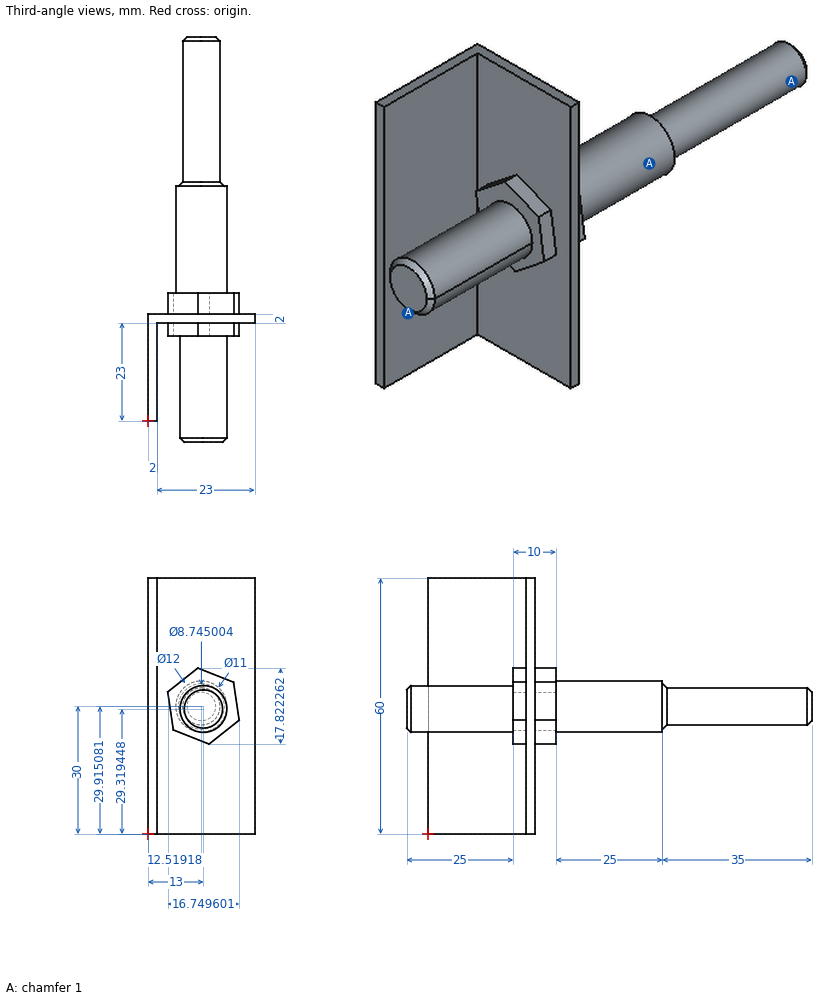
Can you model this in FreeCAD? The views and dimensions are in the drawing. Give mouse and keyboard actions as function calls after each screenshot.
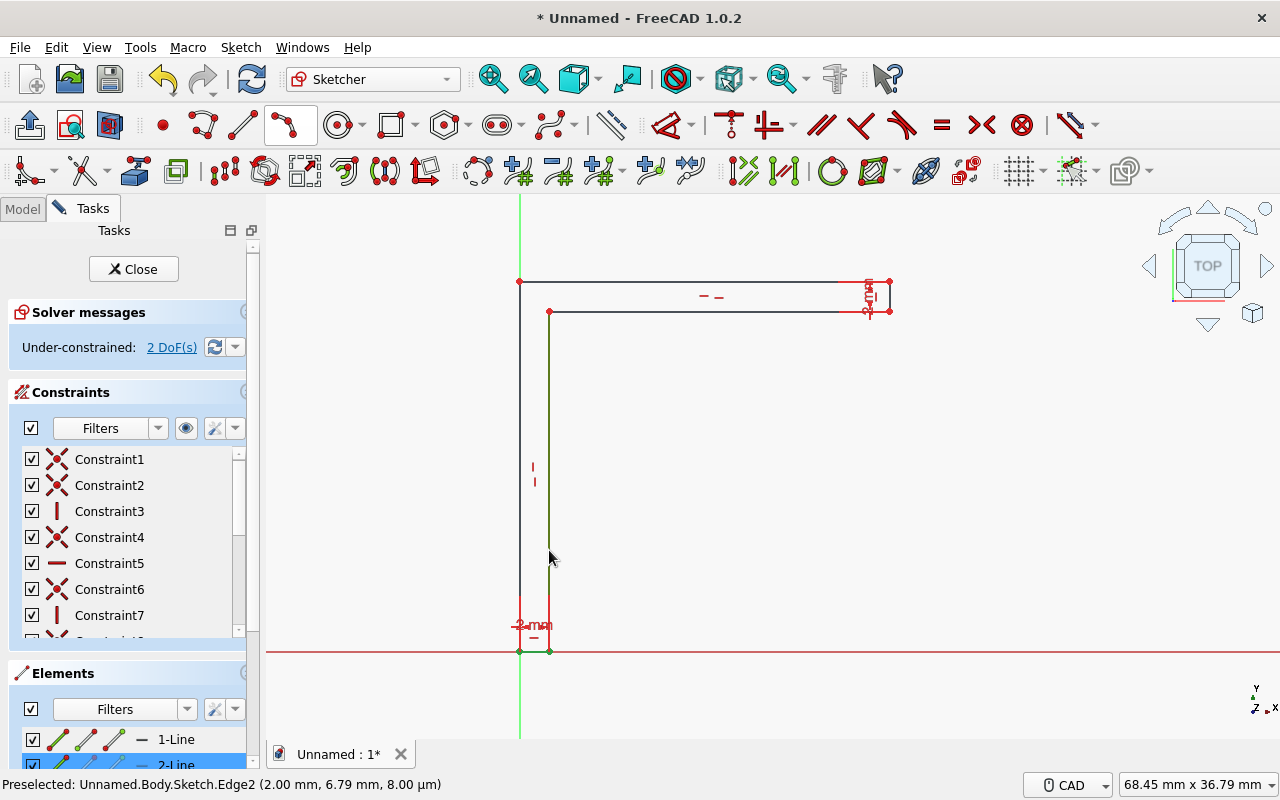
key(i)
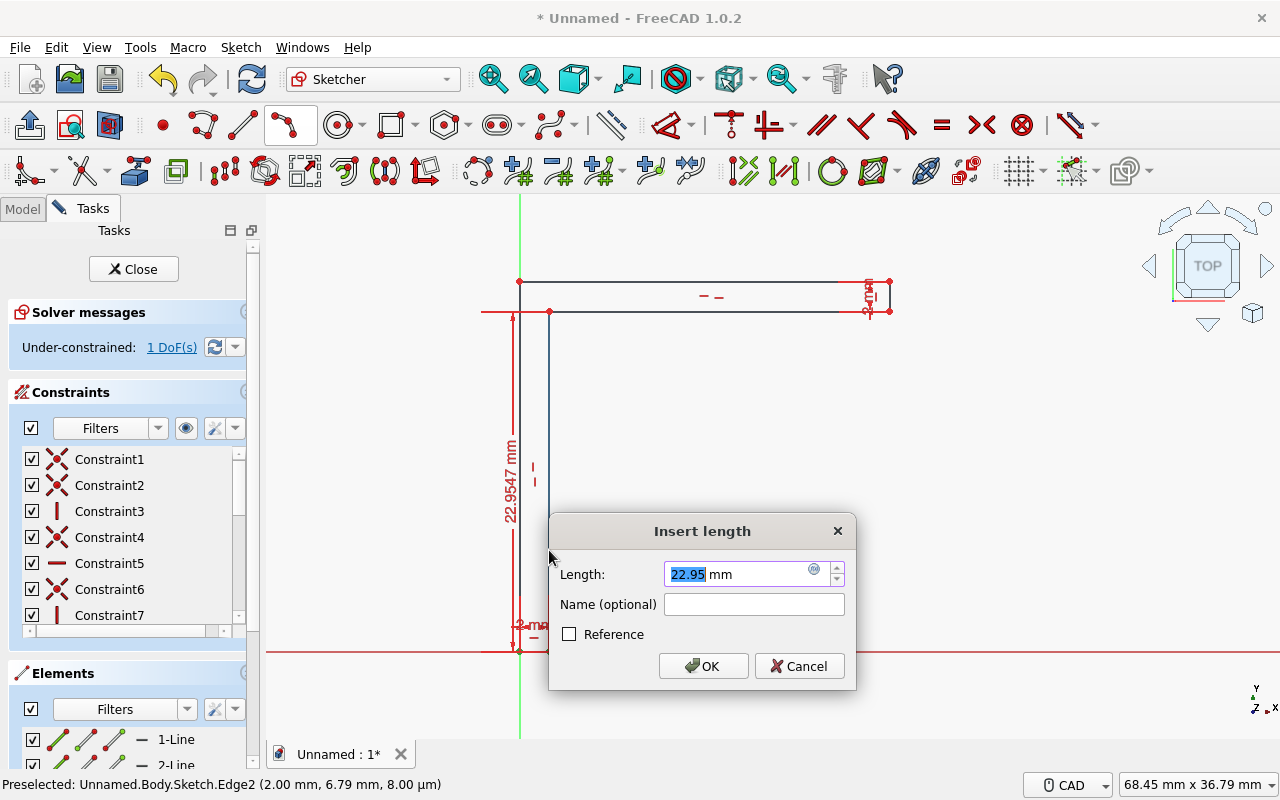
text(23)
key(Return)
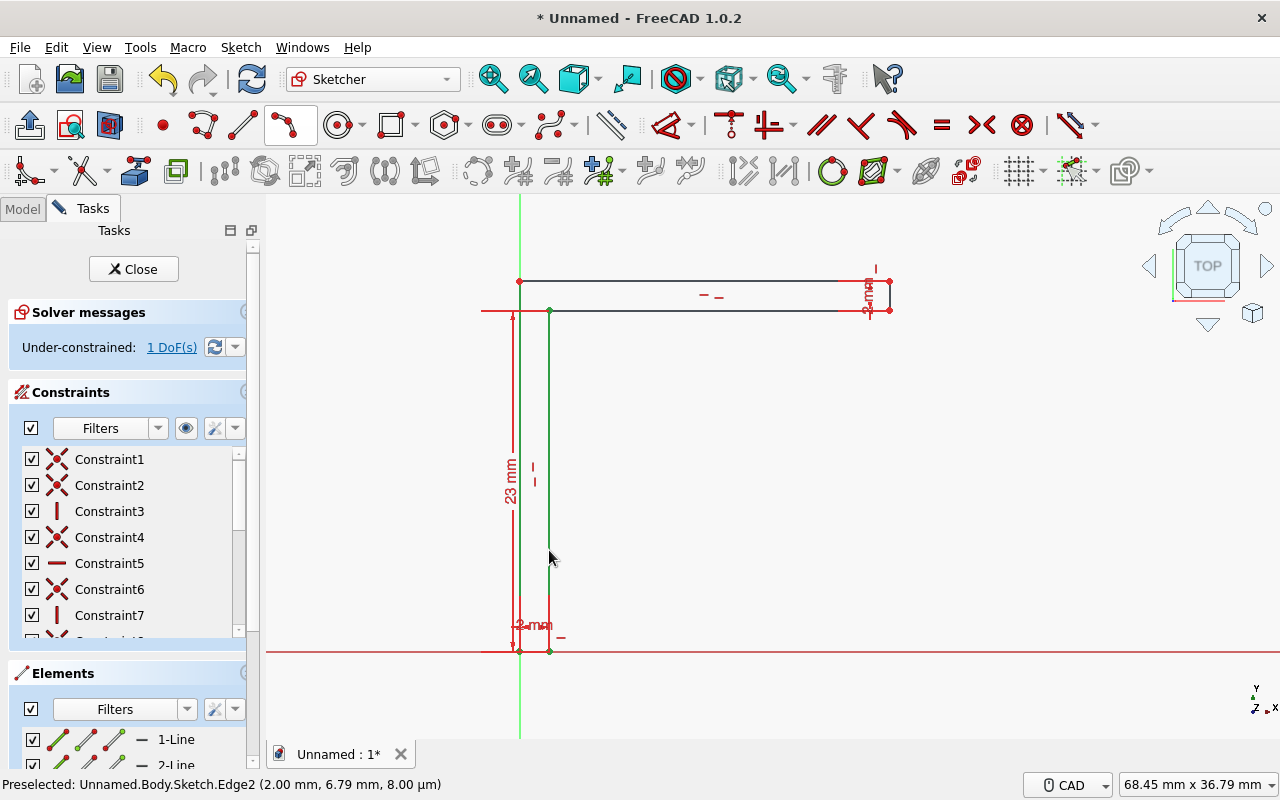
click(651, 311)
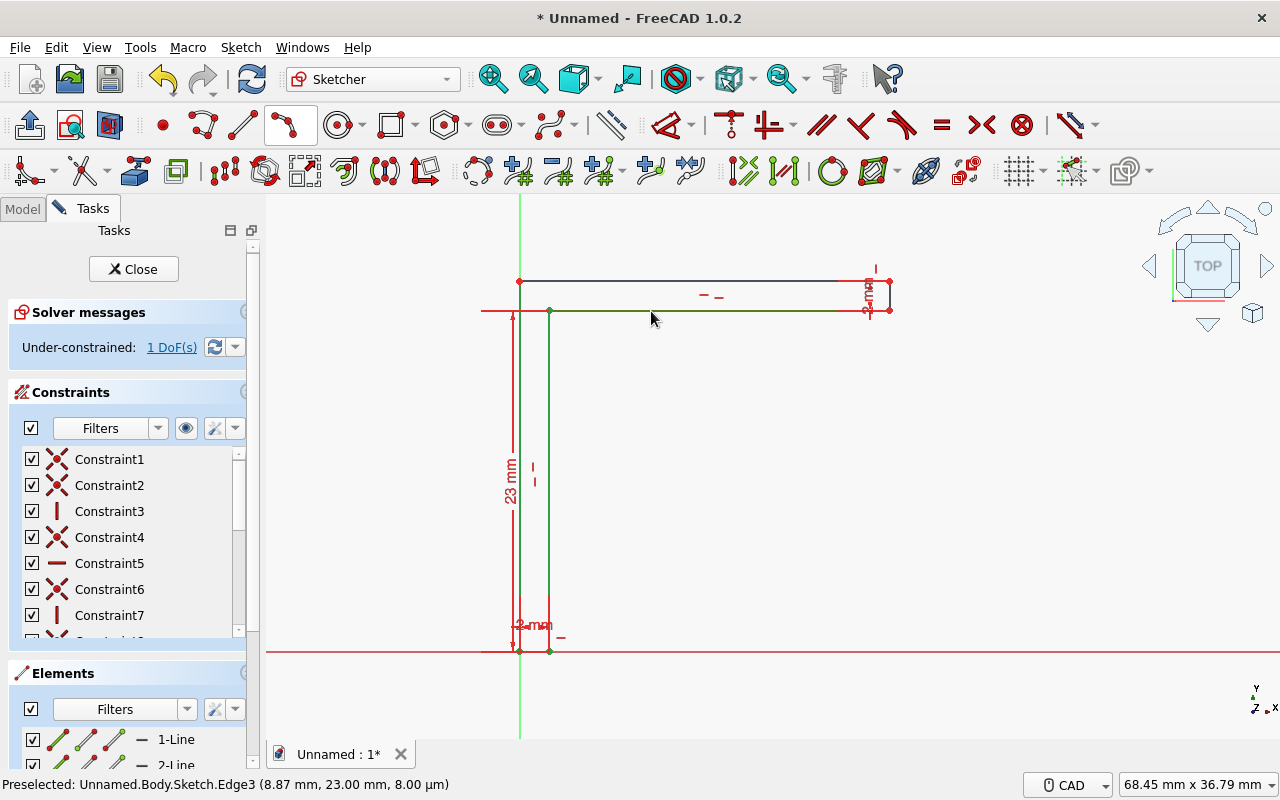
click(694, 126)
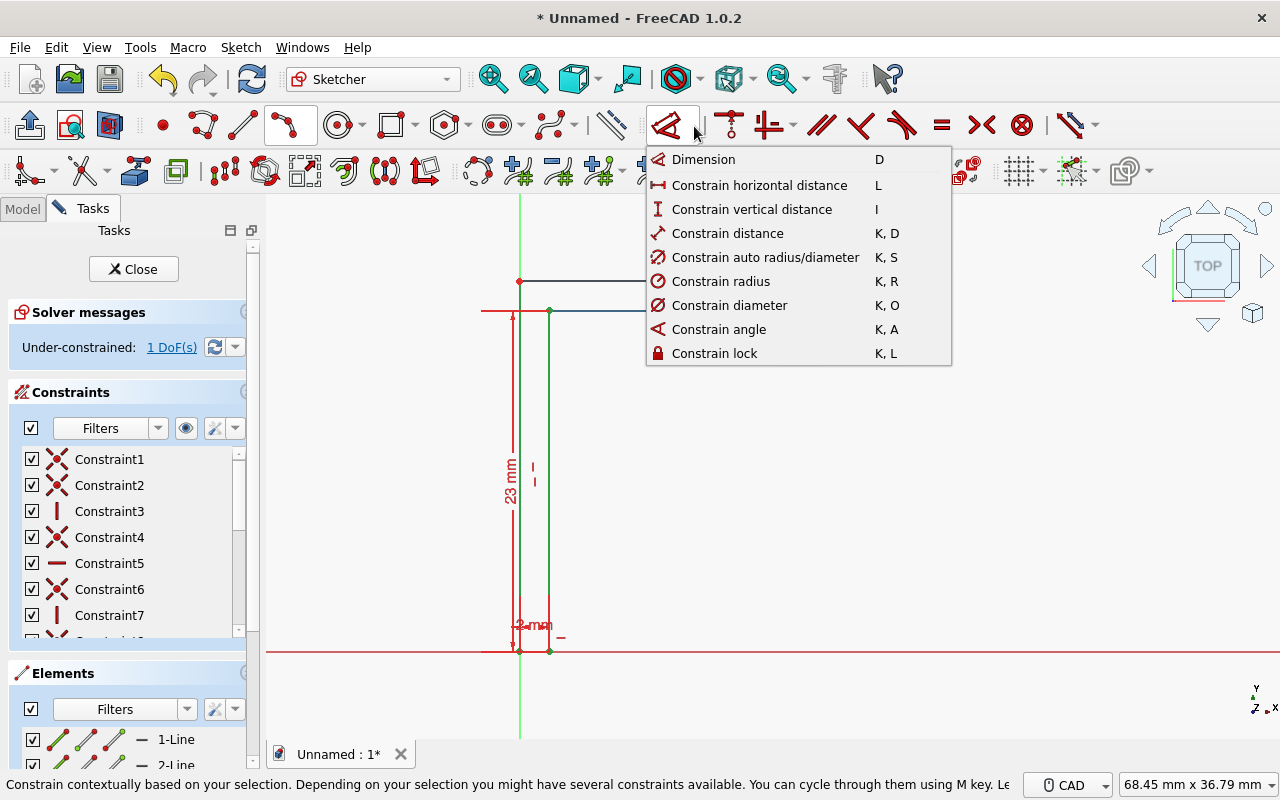
click(799, 185)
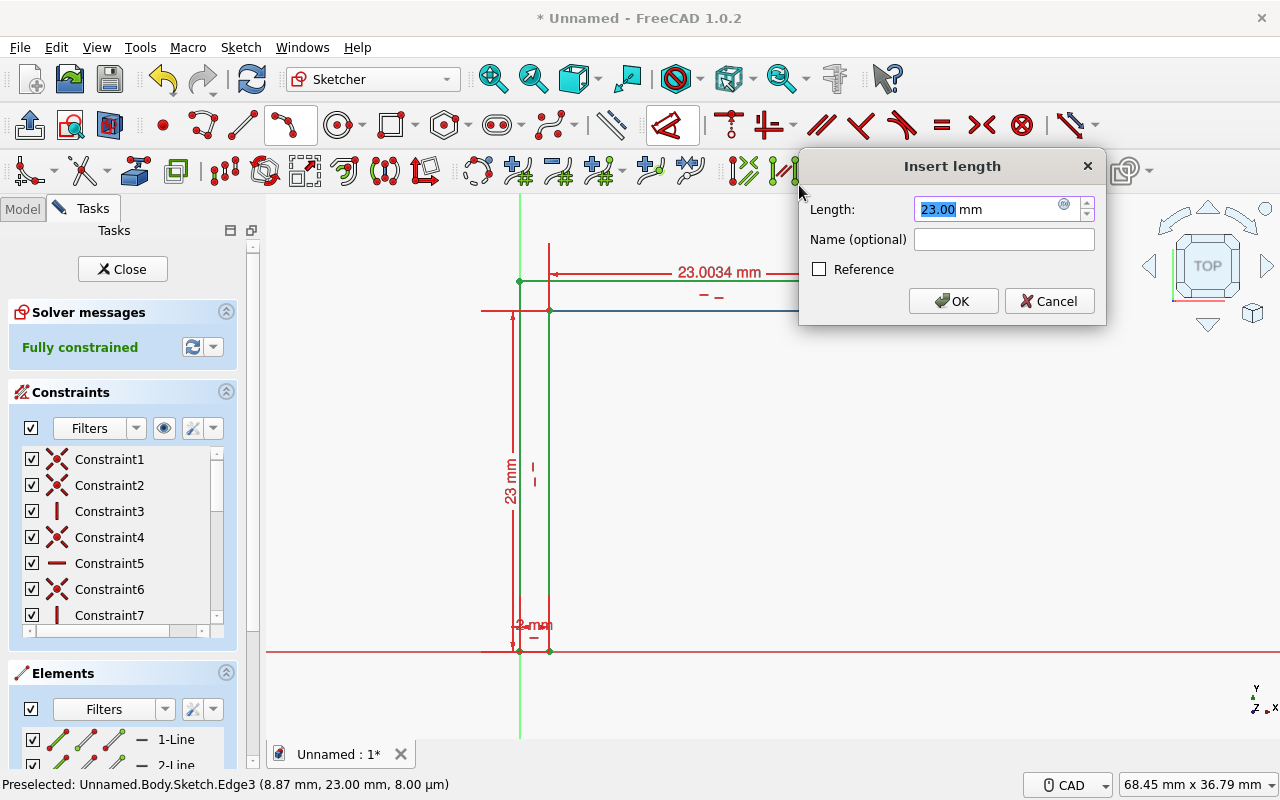
text(23)
key(Return)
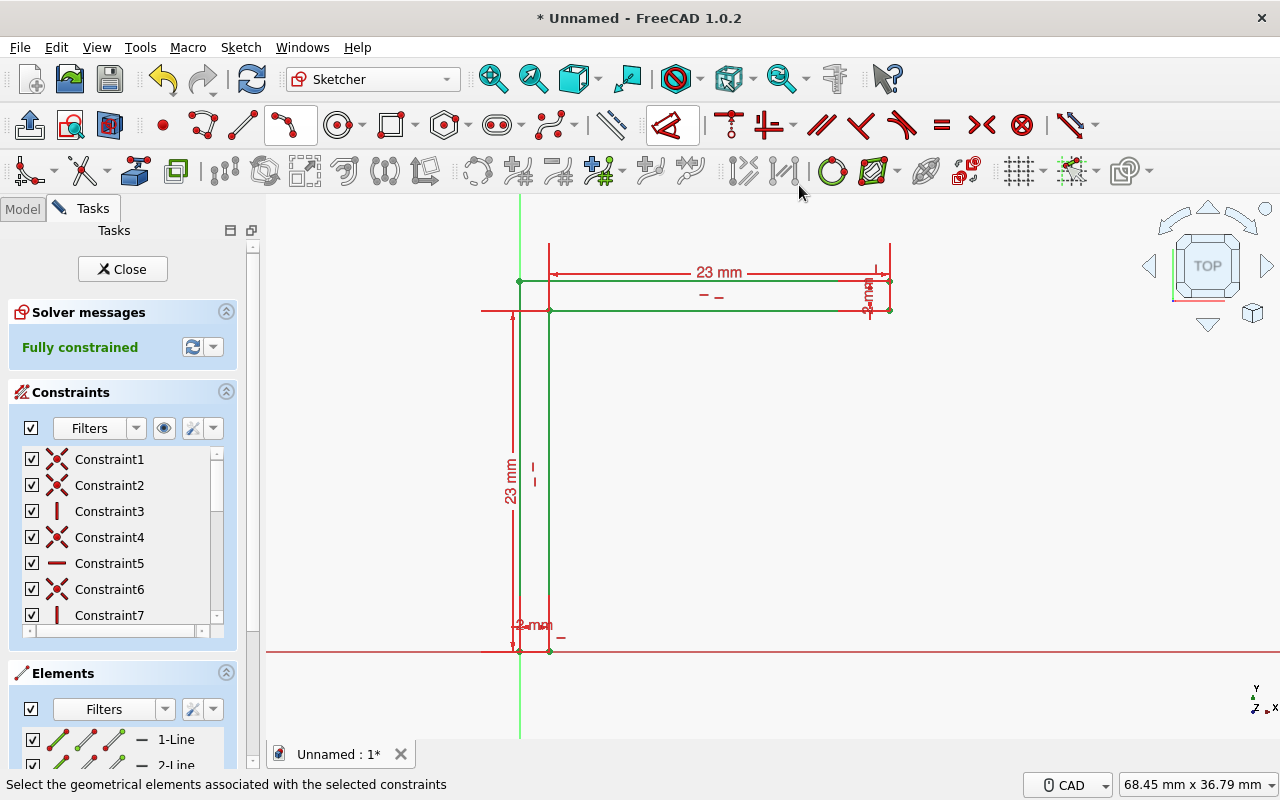
click(123, 269)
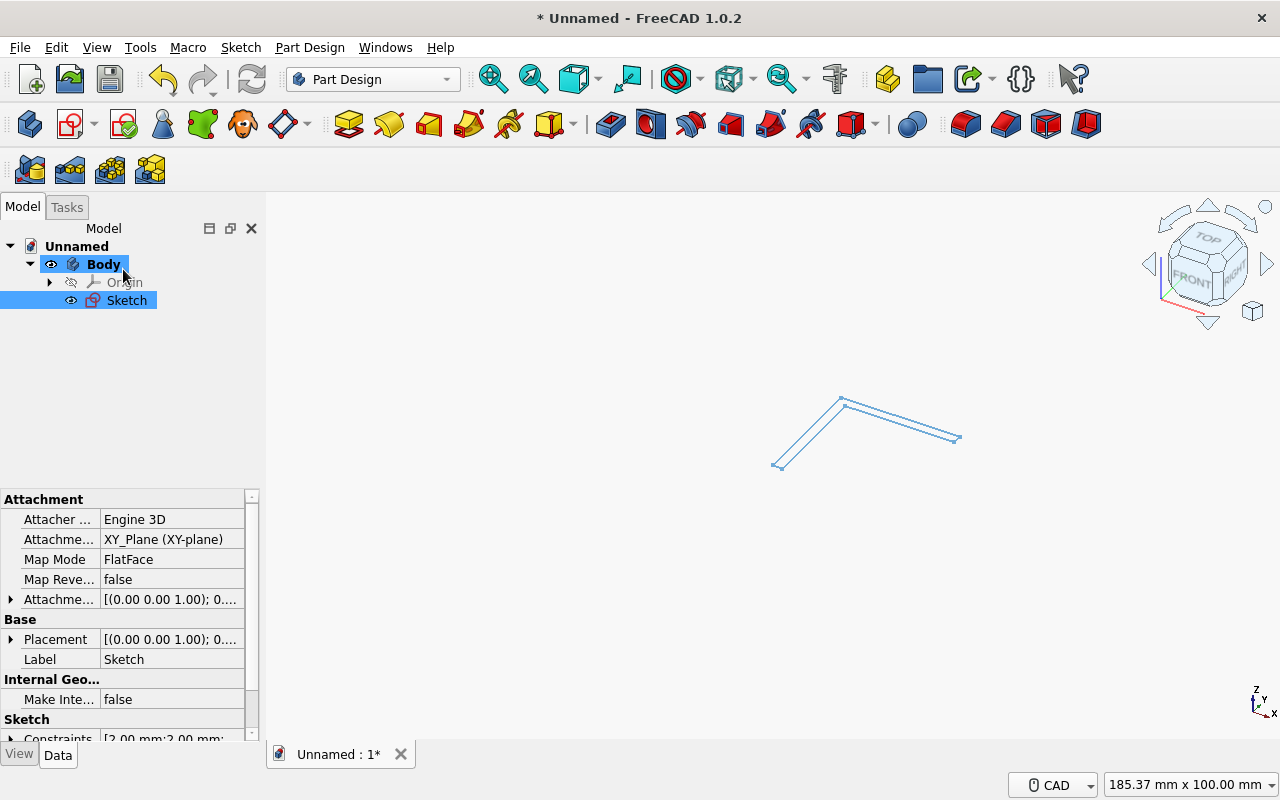
click(350, 124)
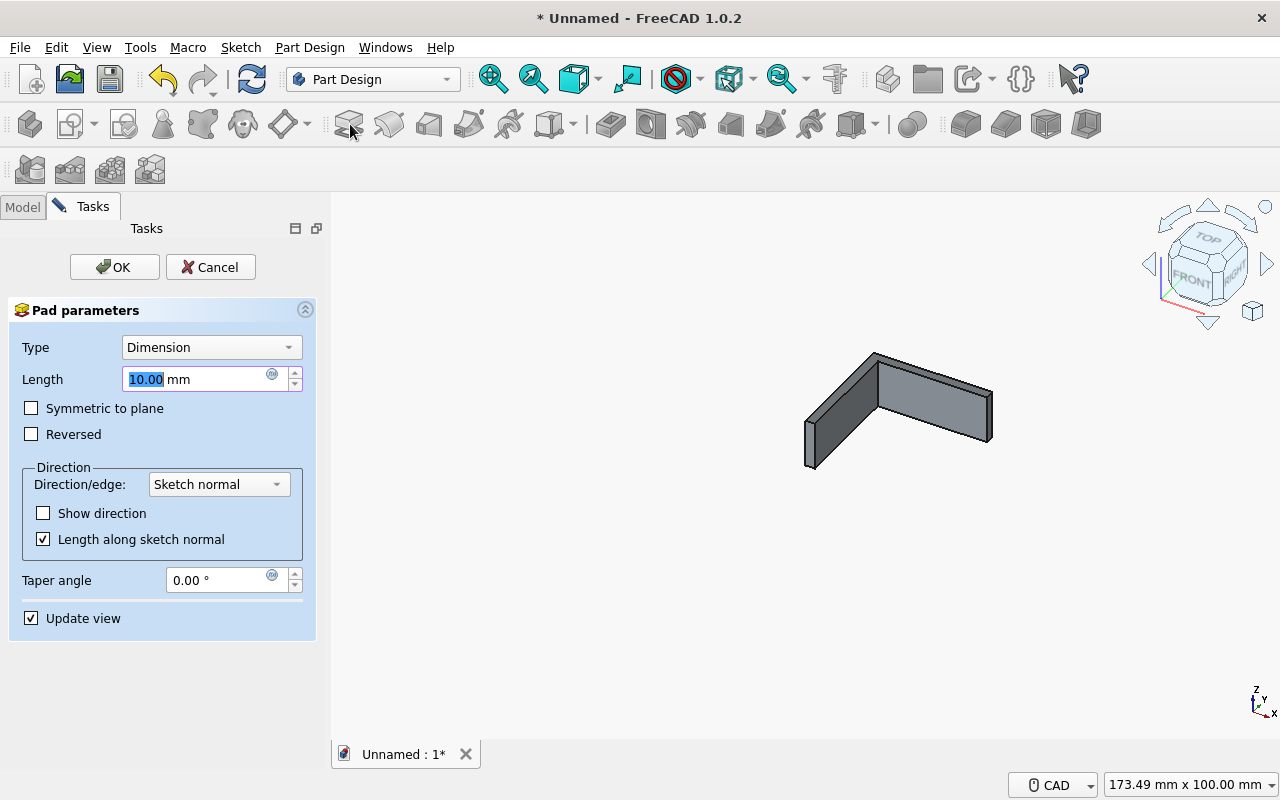
text(60)
key(Tab)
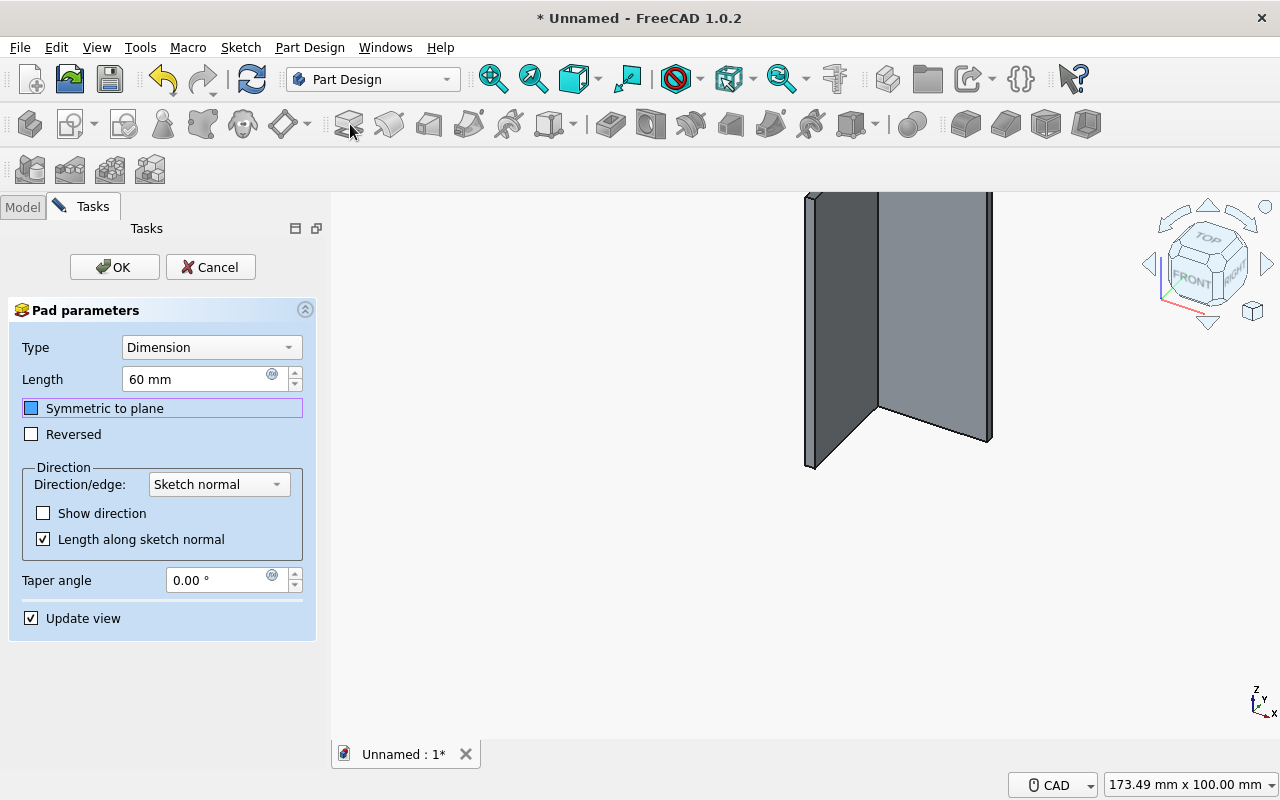
click(115, 267)